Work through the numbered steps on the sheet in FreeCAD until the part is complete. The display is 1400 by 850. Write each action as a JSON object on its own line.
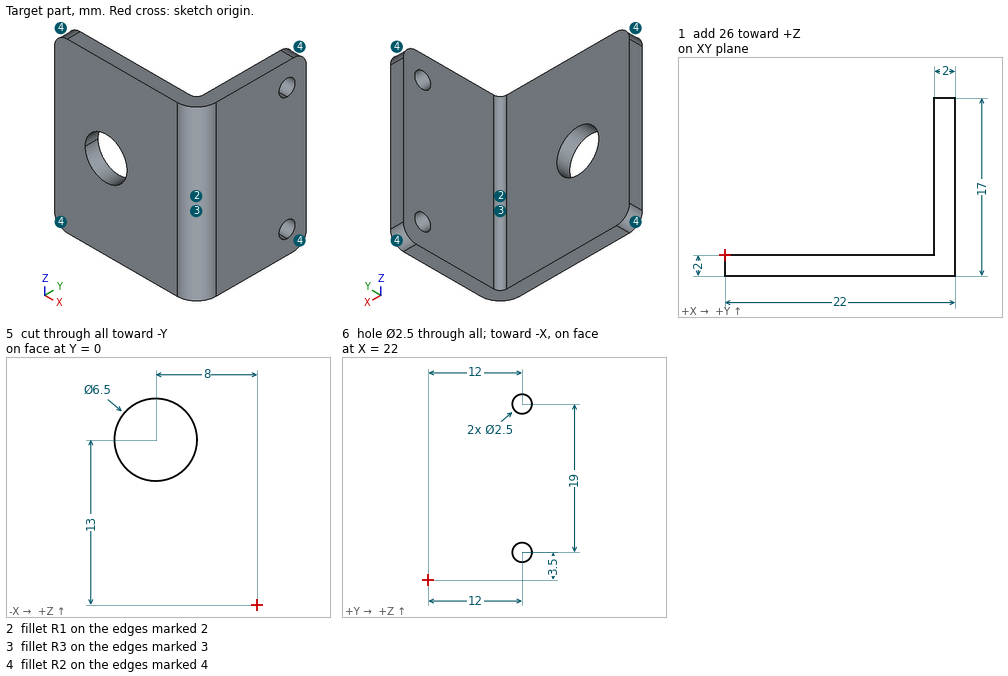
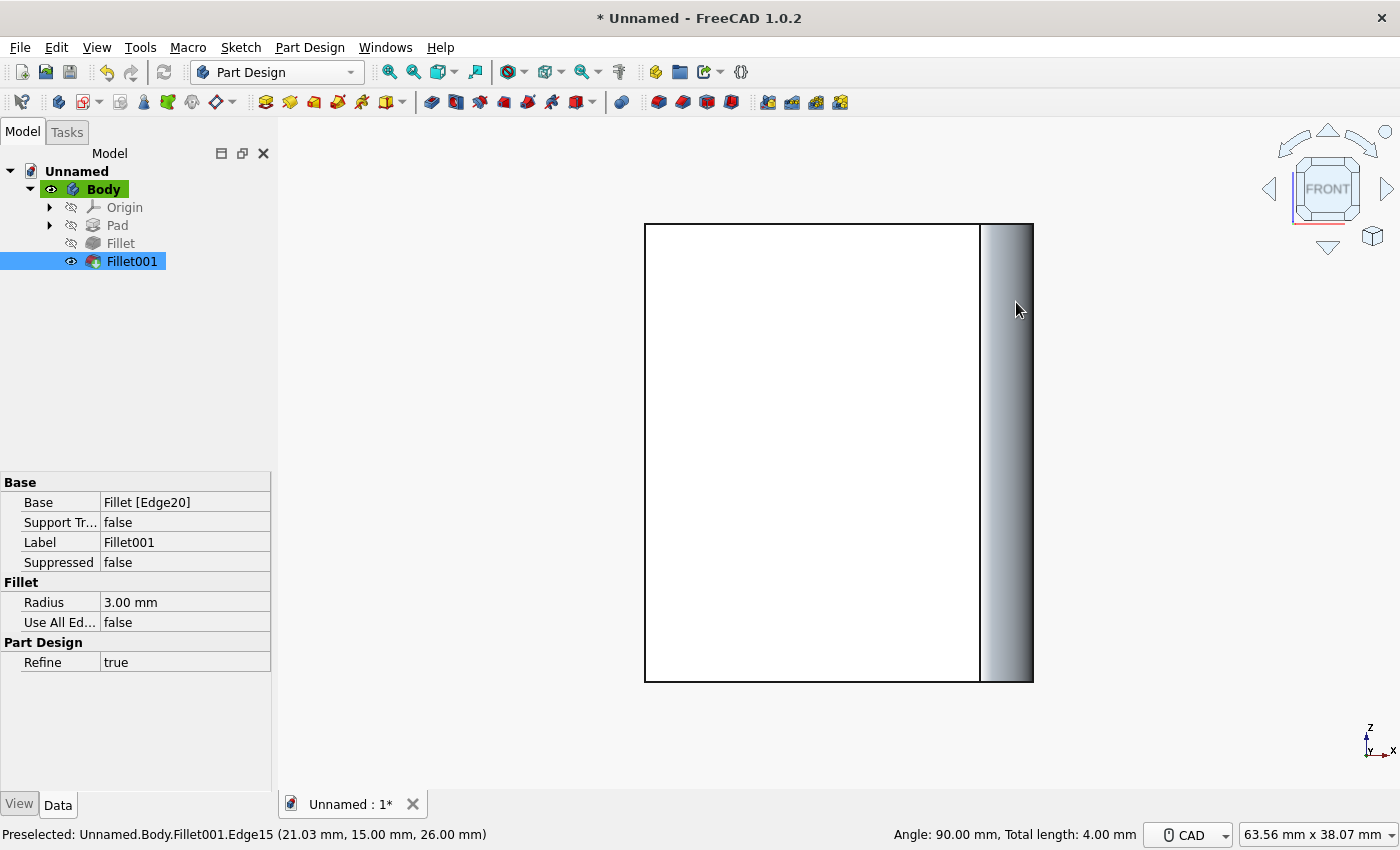
{"action": "key", "text": "3"}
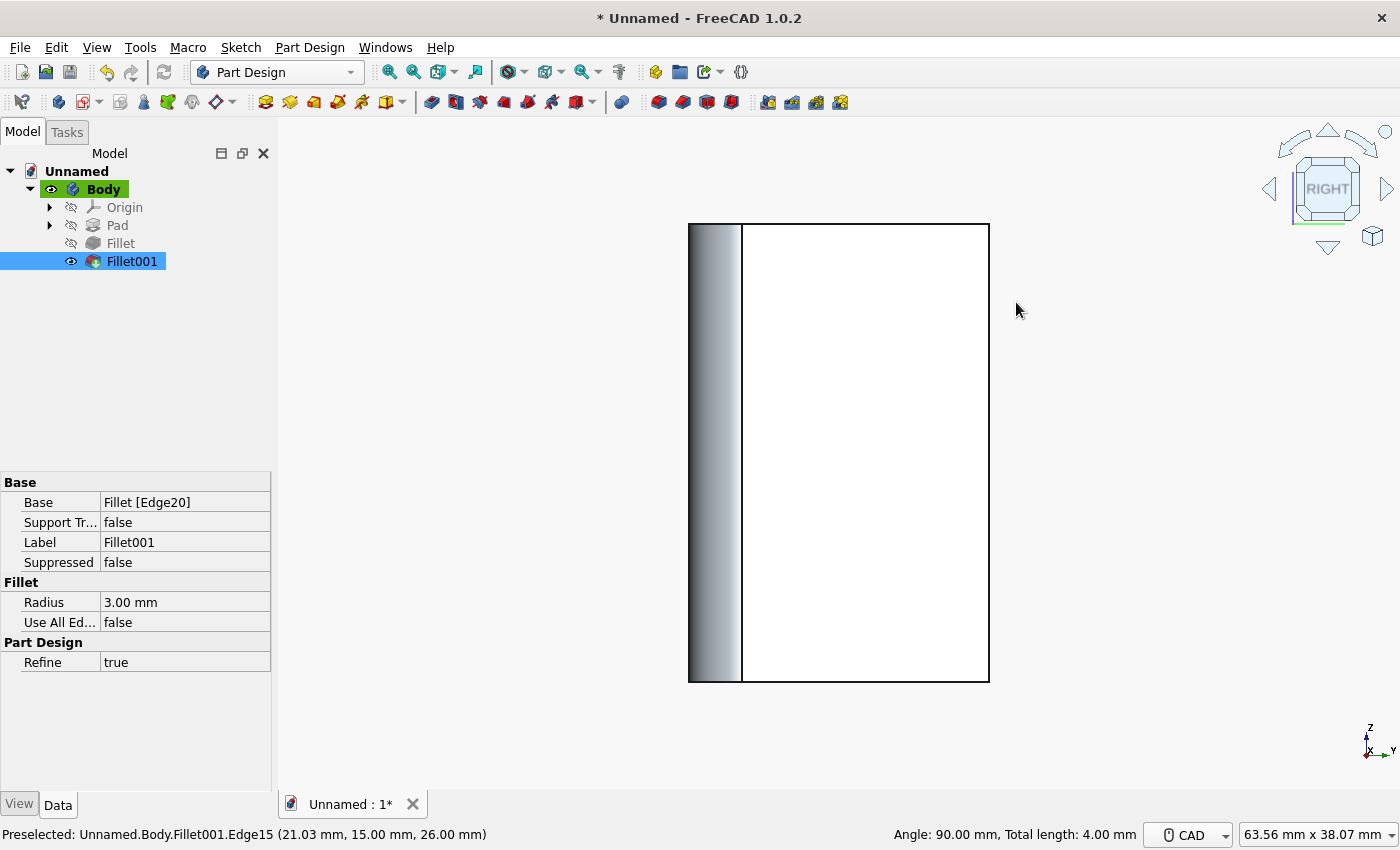
{"action": "key", "text": "5"}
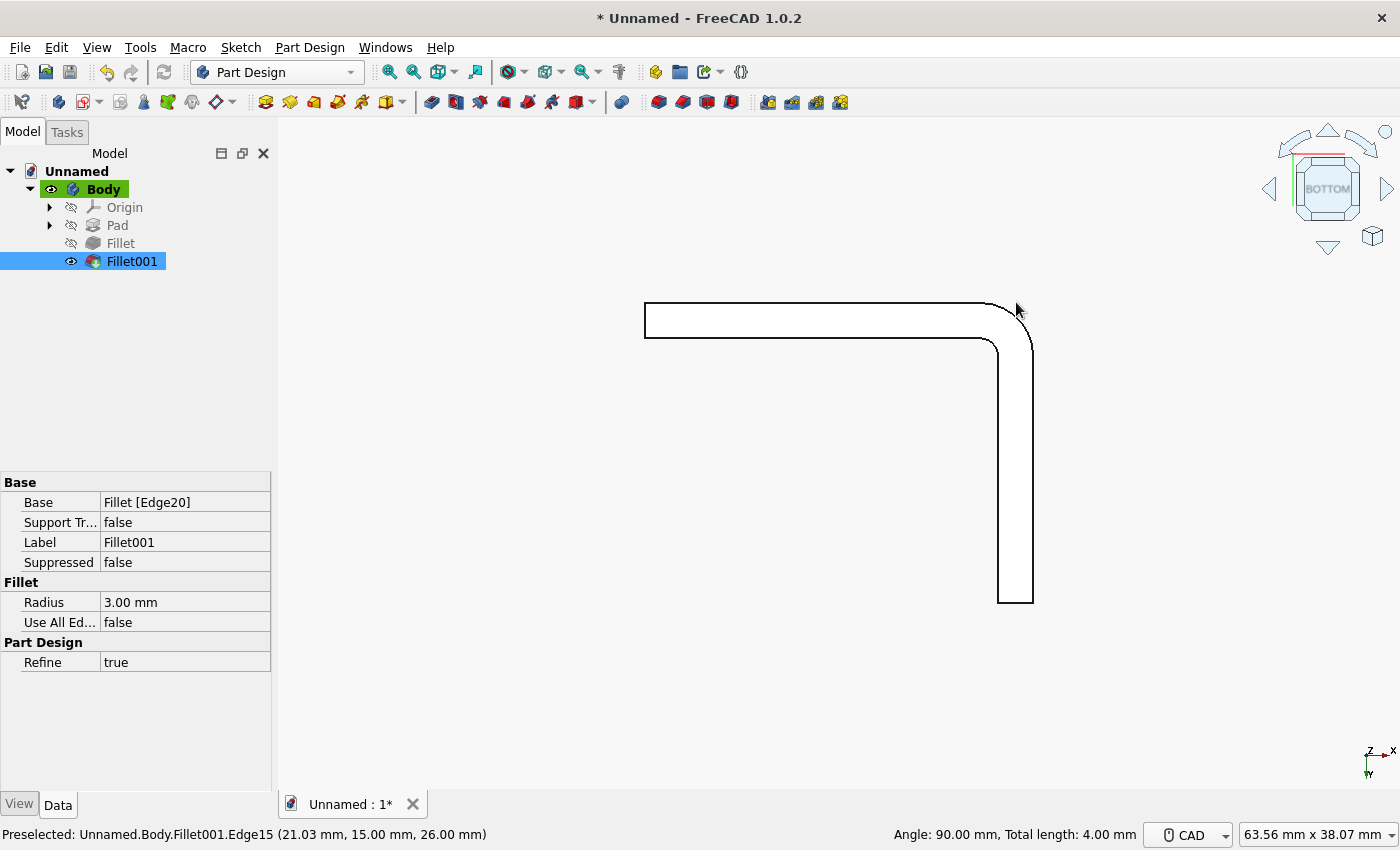
{"action": "key", "text": "v f"}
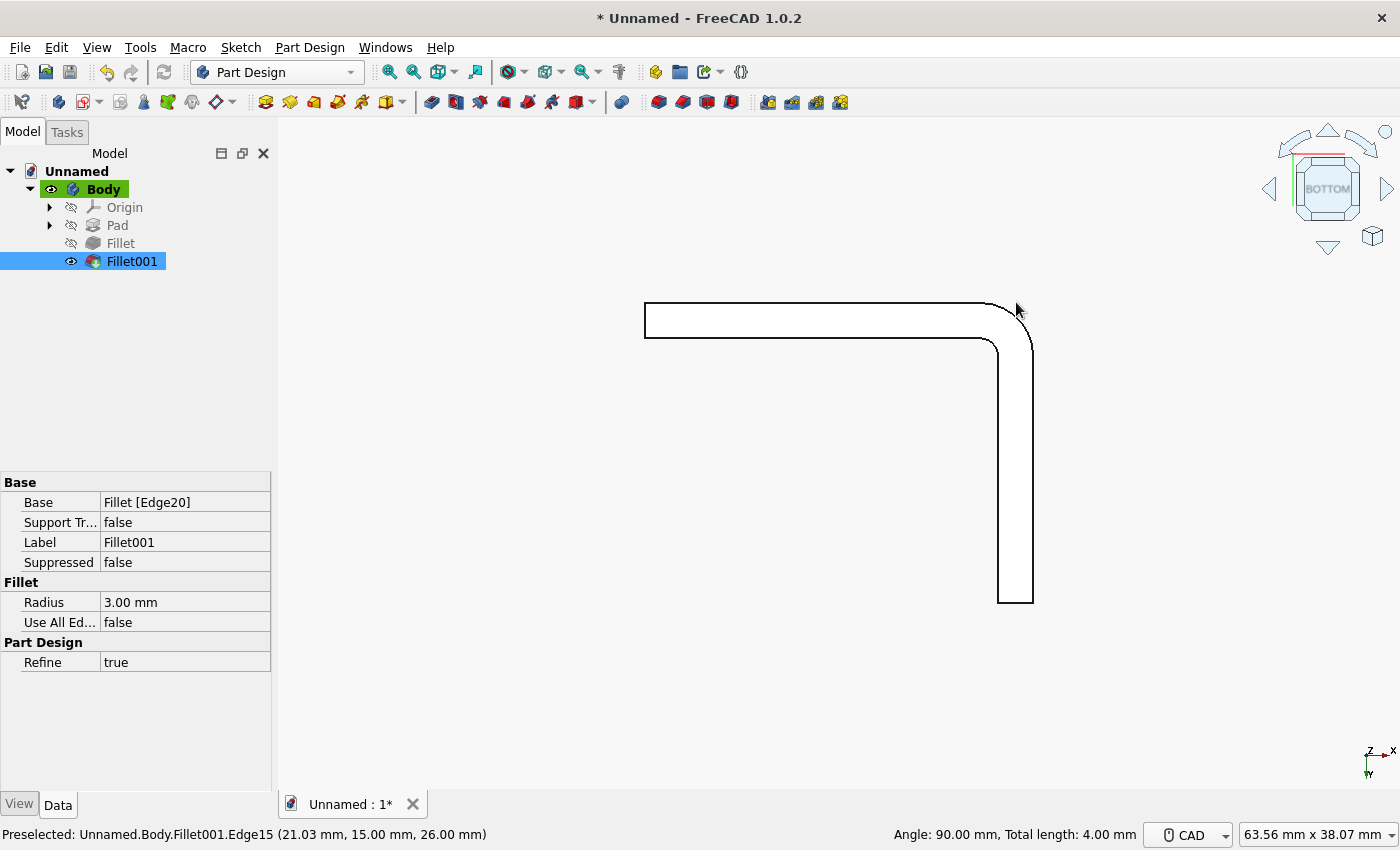
{"action": "left_click", "coordinate": [645, 320], "text": "ctrl"}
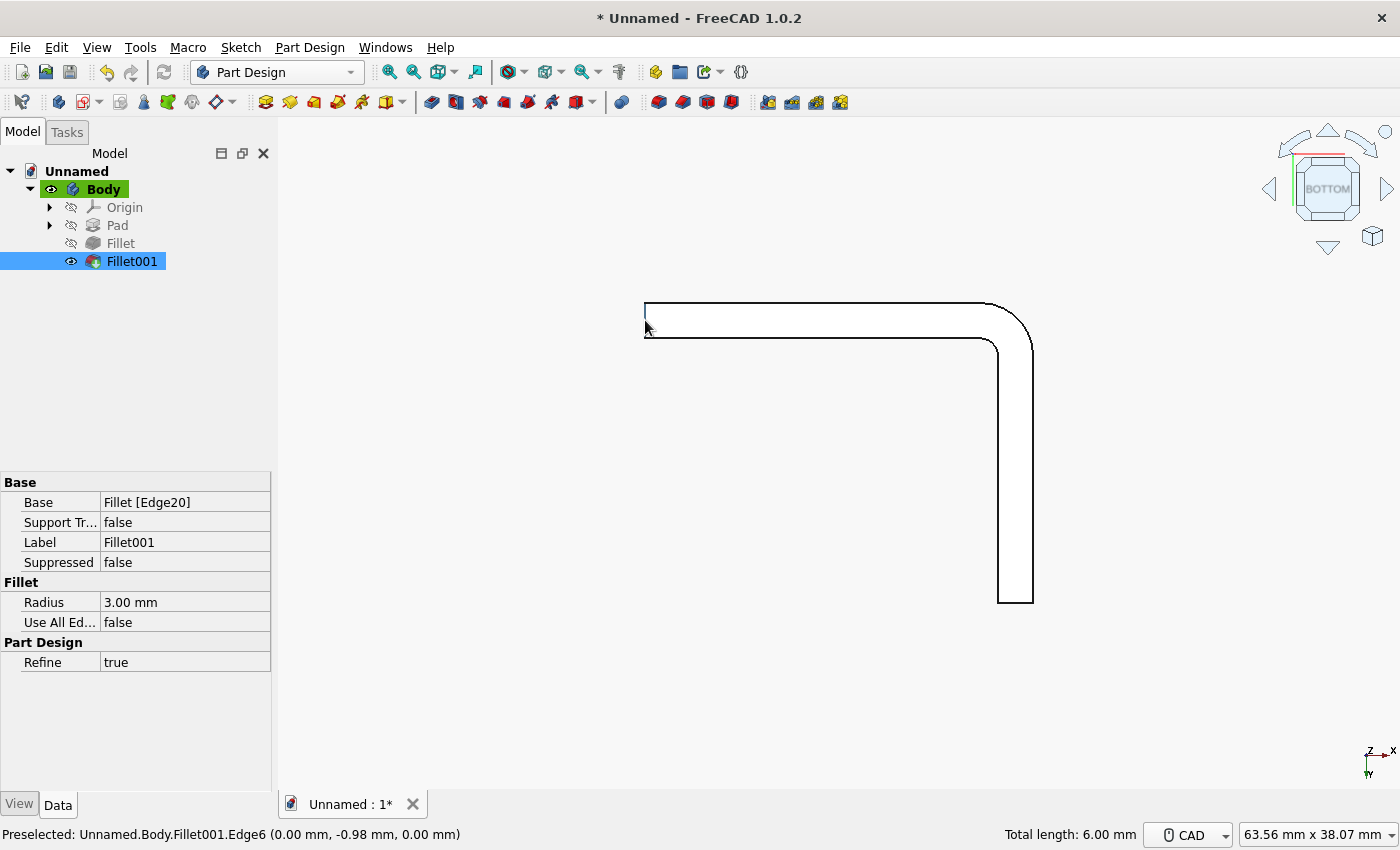
{"action": "left_click", "coordinate": [1016, 602], "text": "ctrl"}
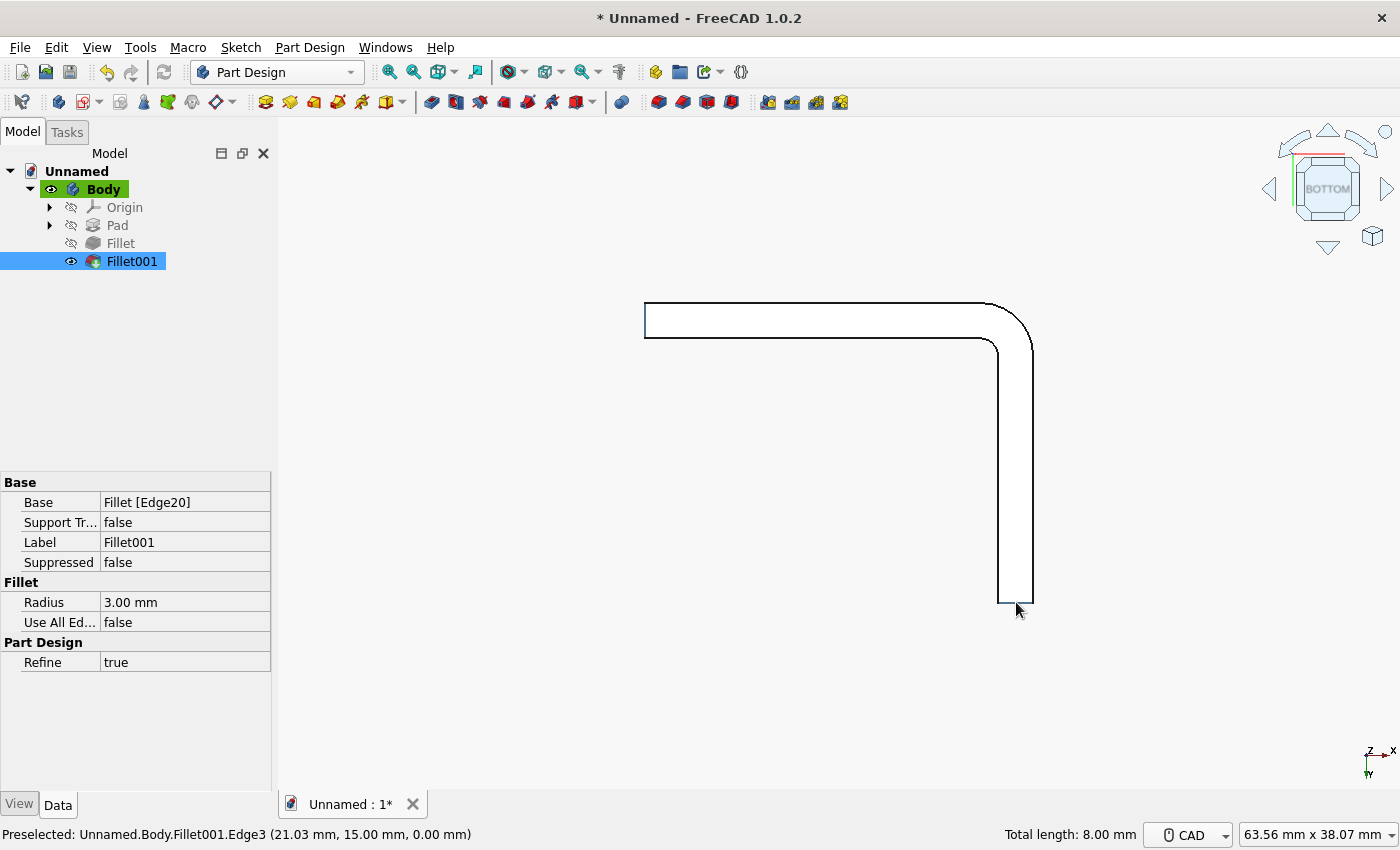
{"action": "left_click", "coordinate": [660, 102]}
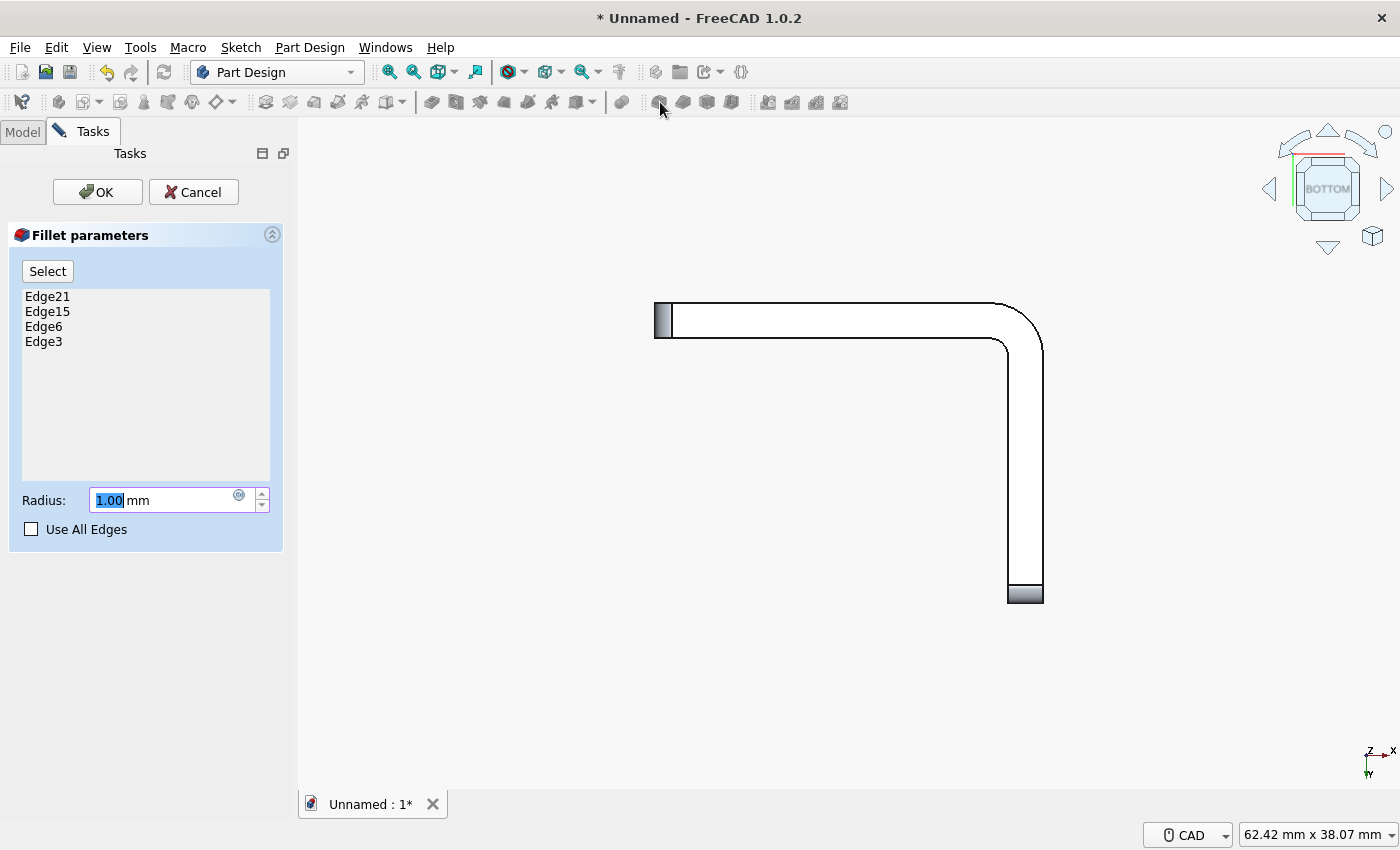
{"action": "type", "text": "2"}
{"action": "key", "text": "Tab"}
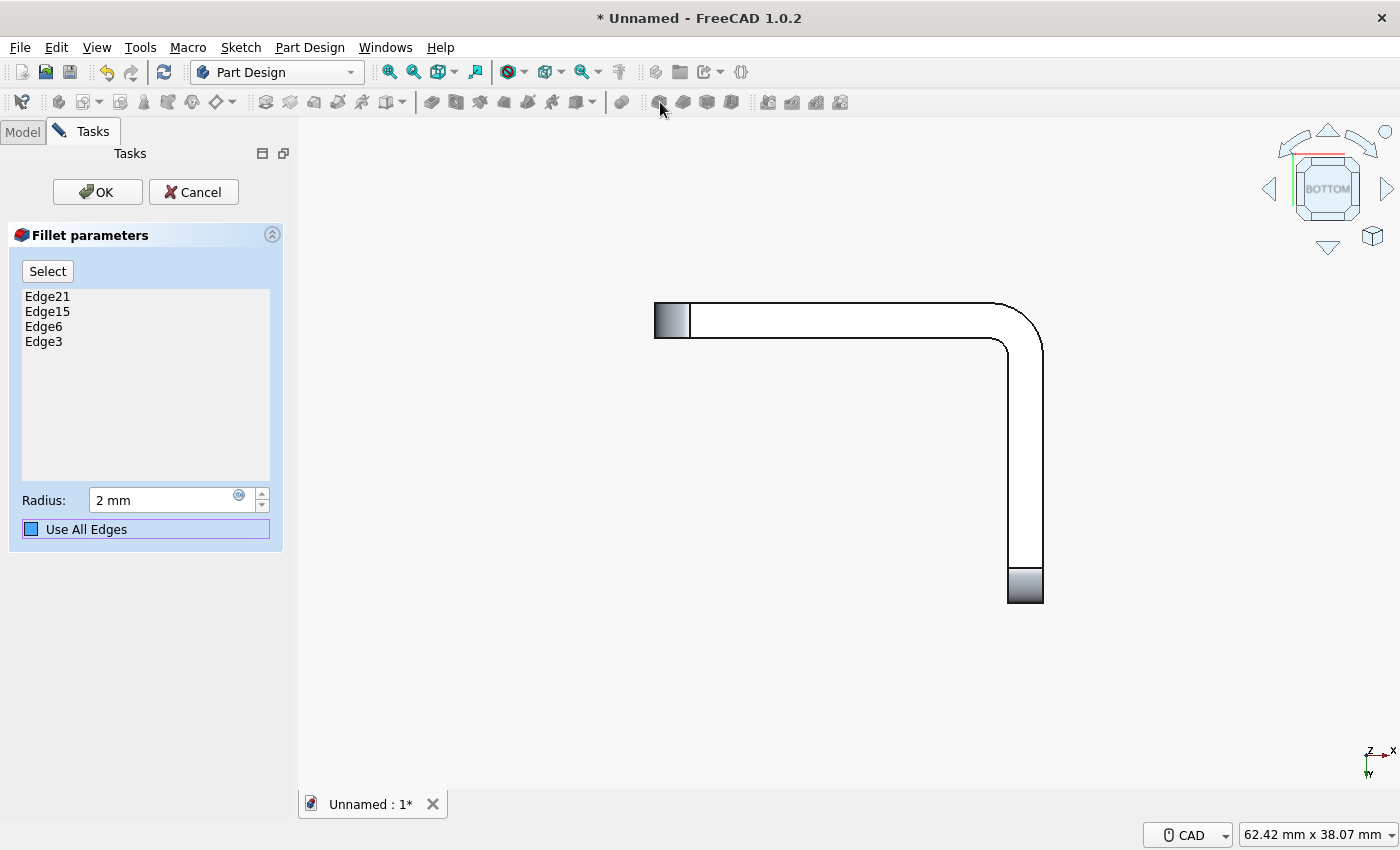
{"action": "left_click", "coordinate": [98, 192]}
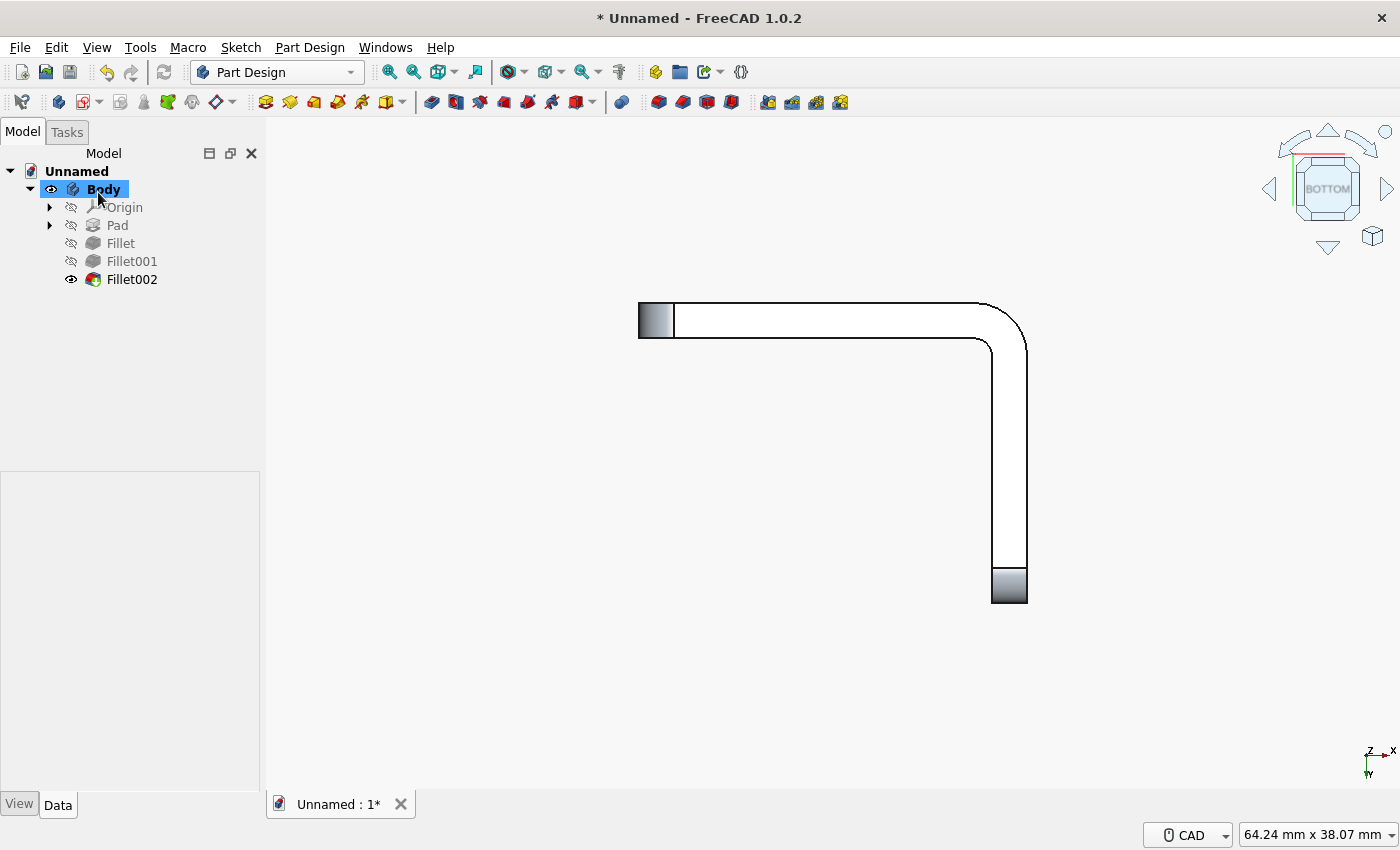
{"action": "key", "text": "v f"}